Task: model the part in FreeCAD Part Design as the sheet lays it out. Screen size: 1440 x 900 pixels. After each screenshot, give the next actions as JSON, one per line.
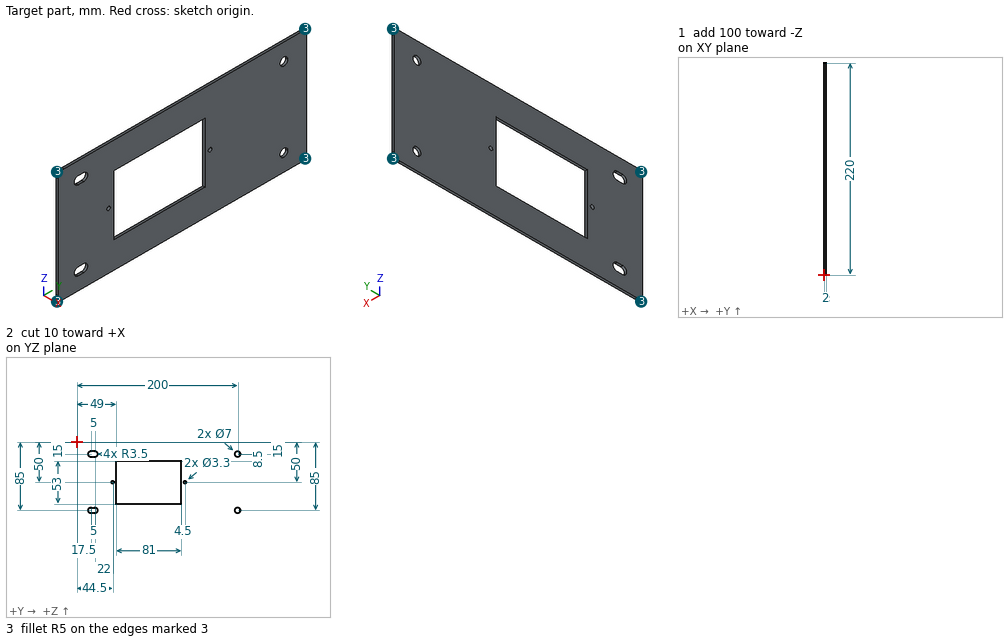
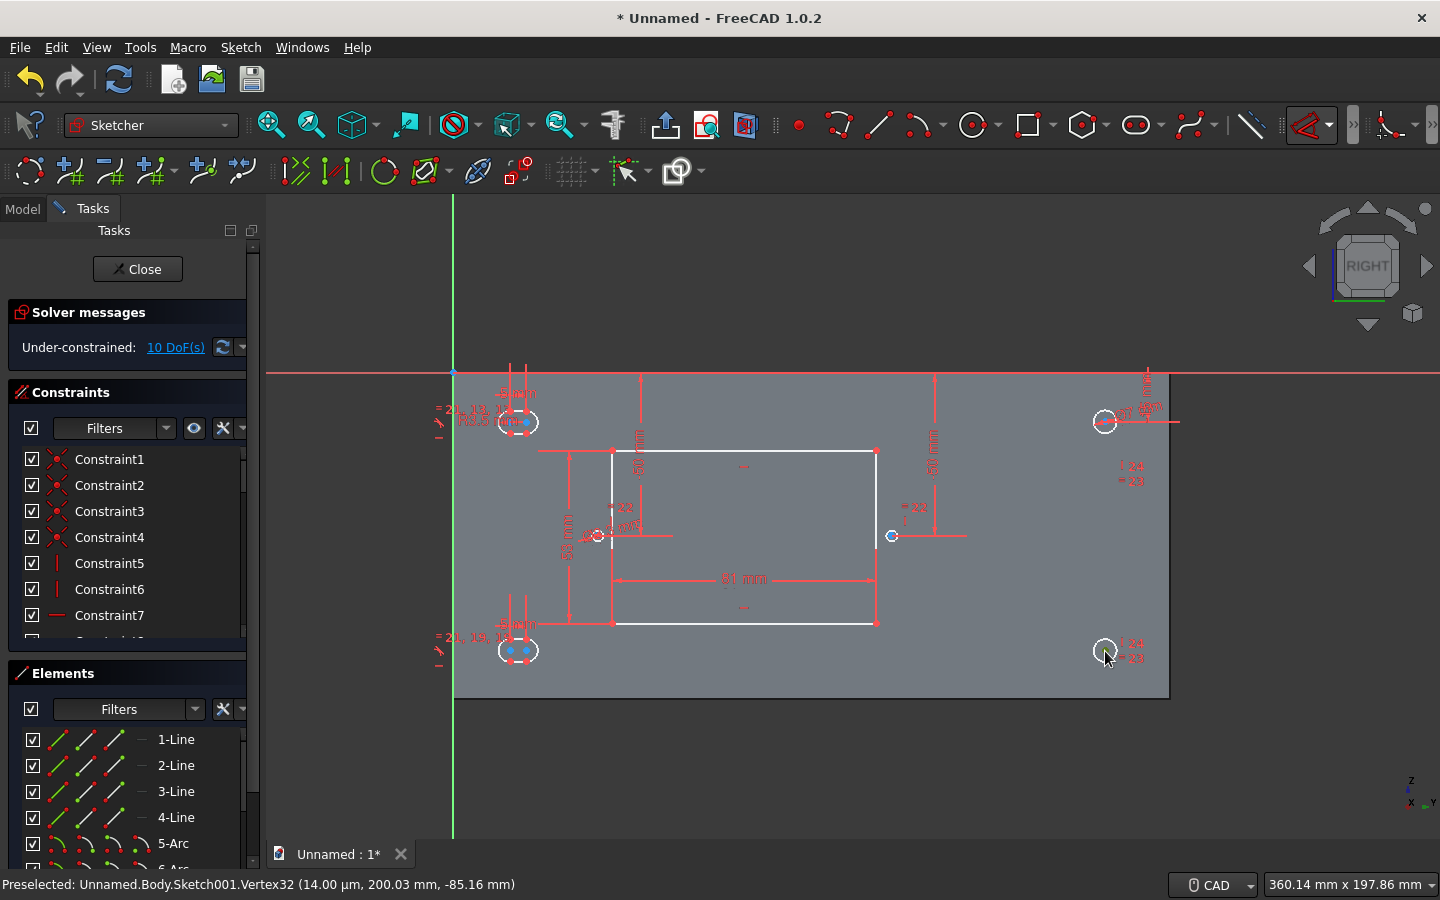
{"action": "key", "text": "i"}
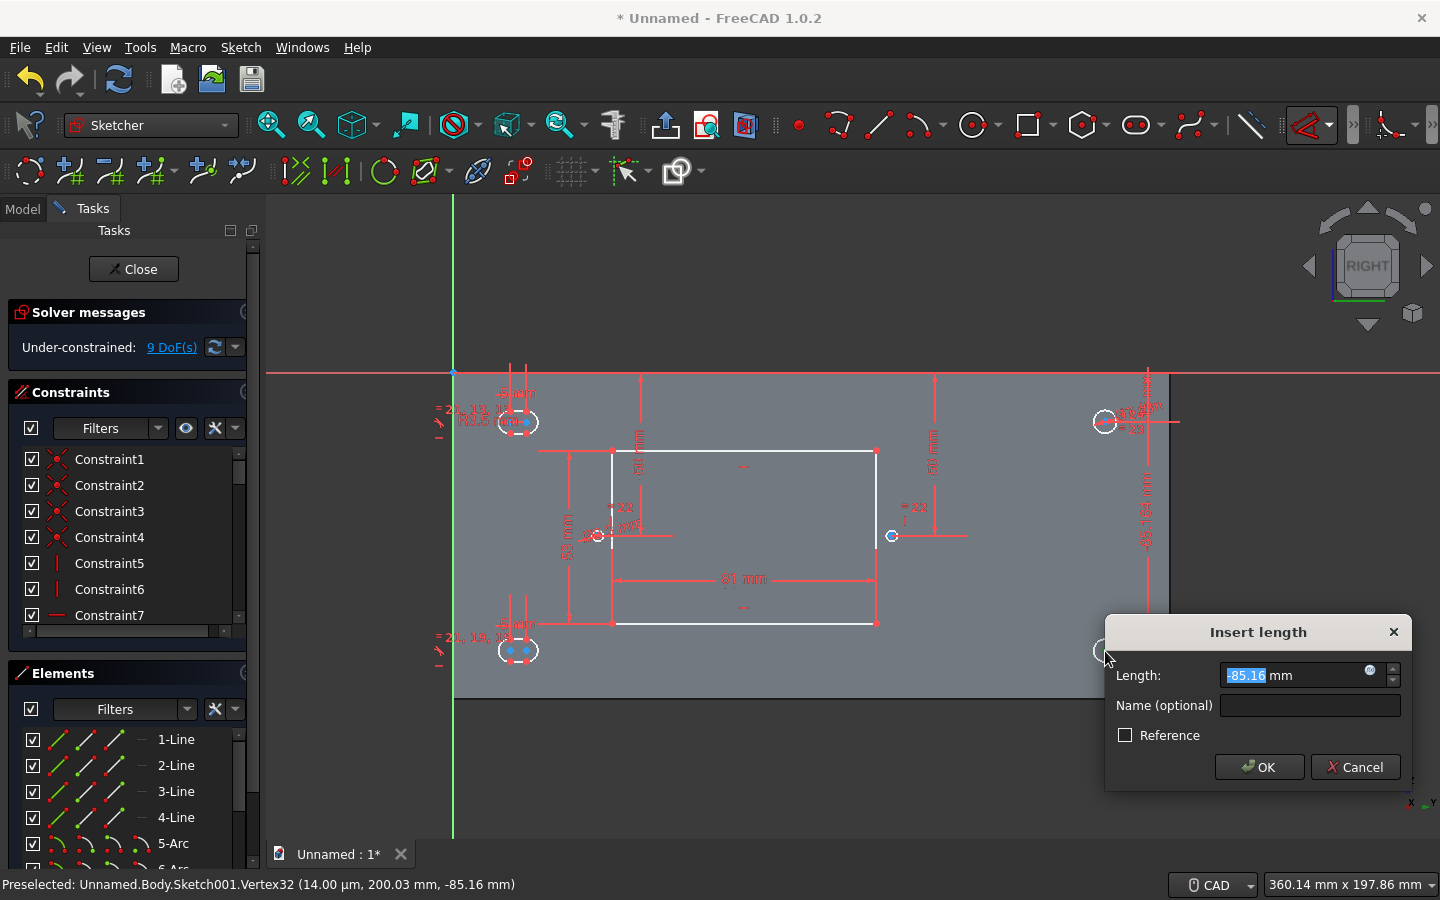
{"action": "type", "text": "-85"}
{"action": "key", "text": "Return"}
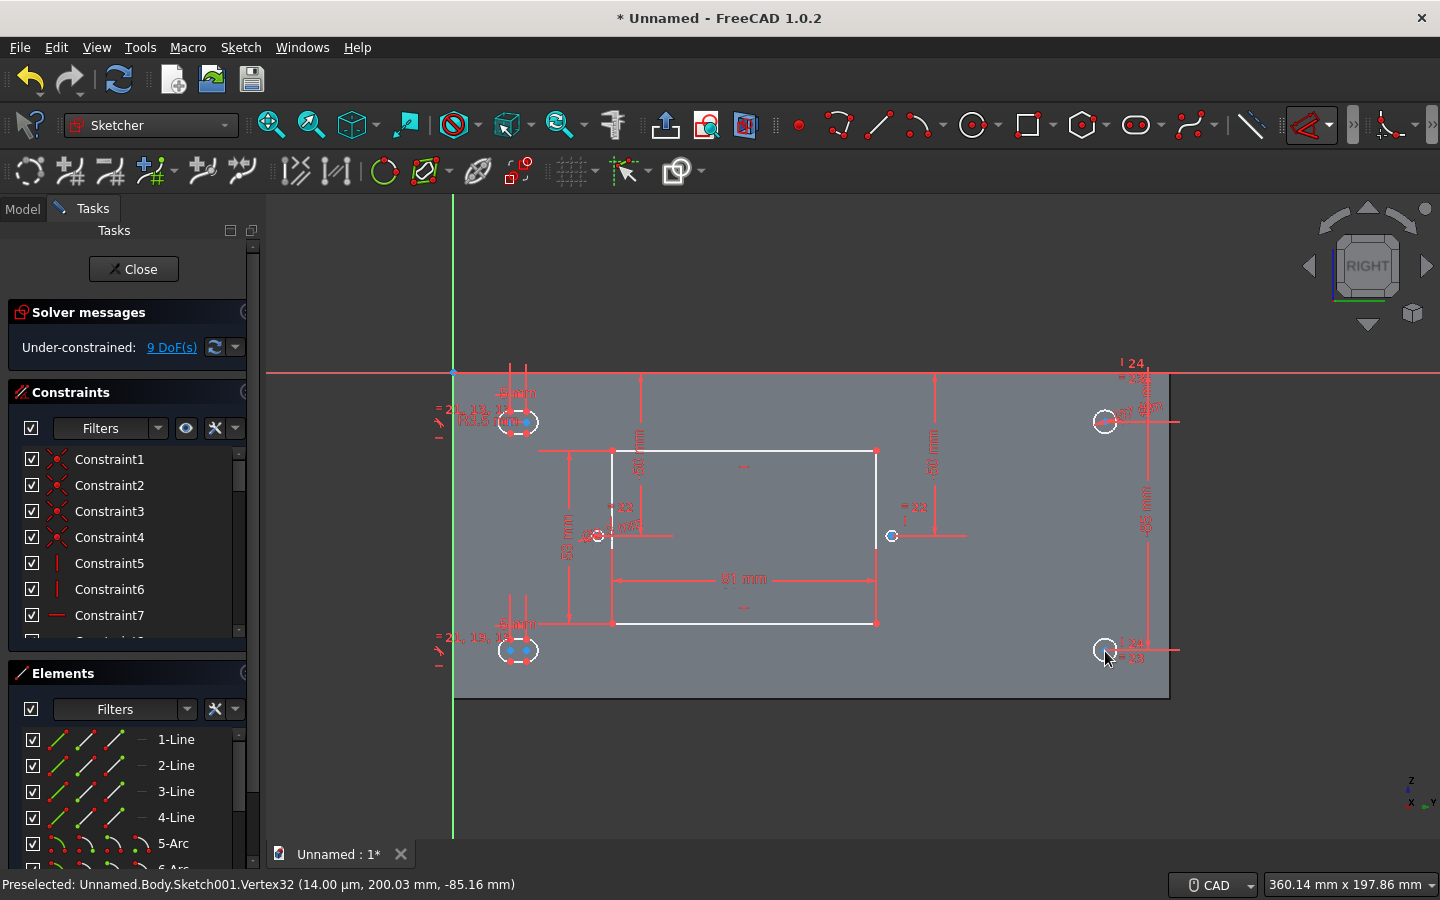
{"action": "left_click", "coordinate": [612, 451]}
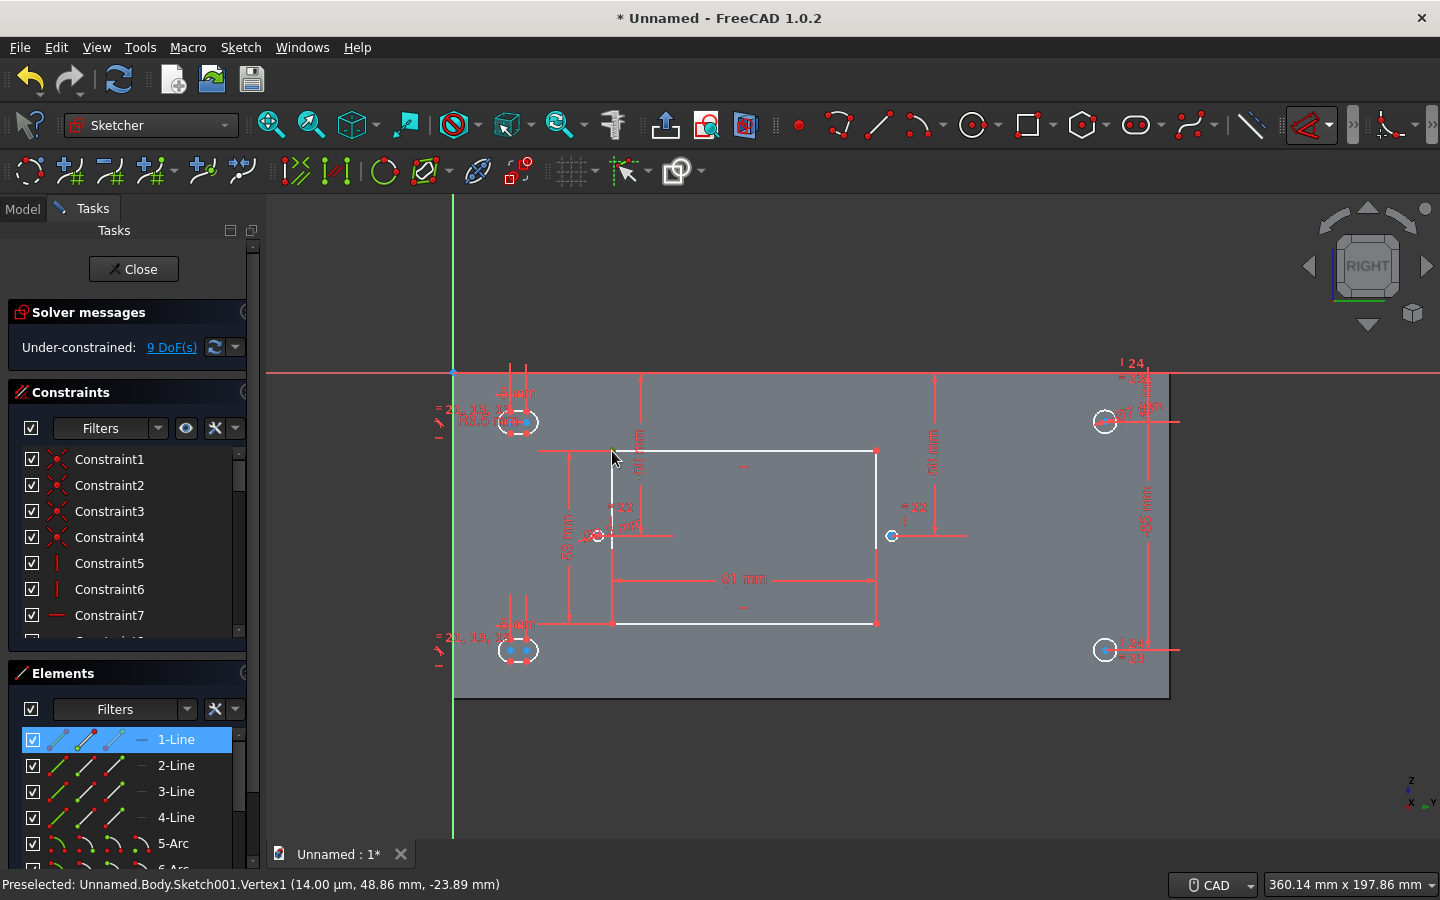
{"action": "left_click", "coordinate": [1332, 126]}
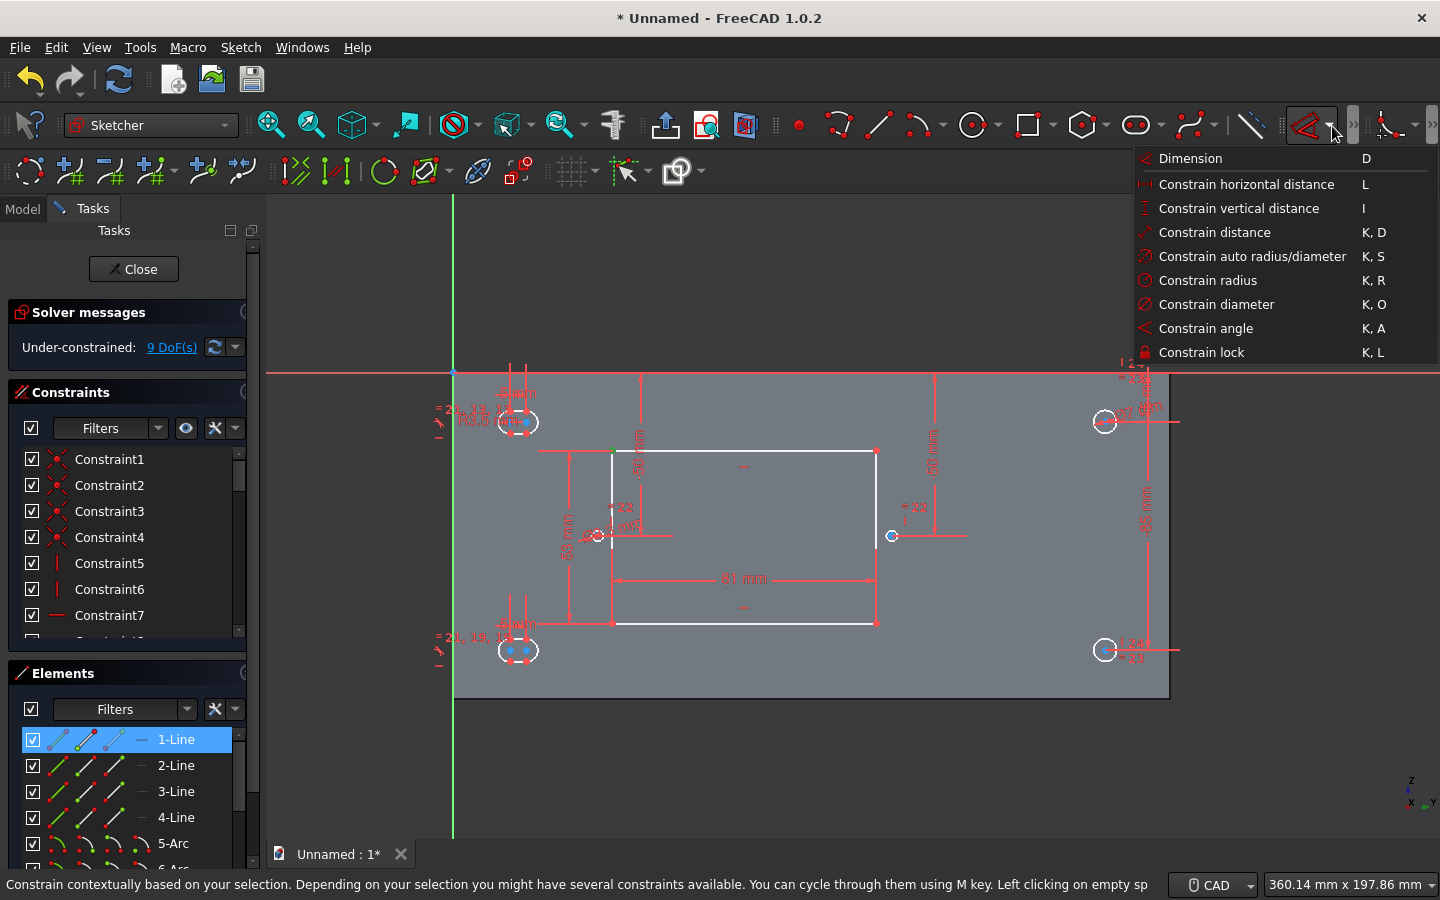
{"action": "left_click", "coordinate": [1286, 184]}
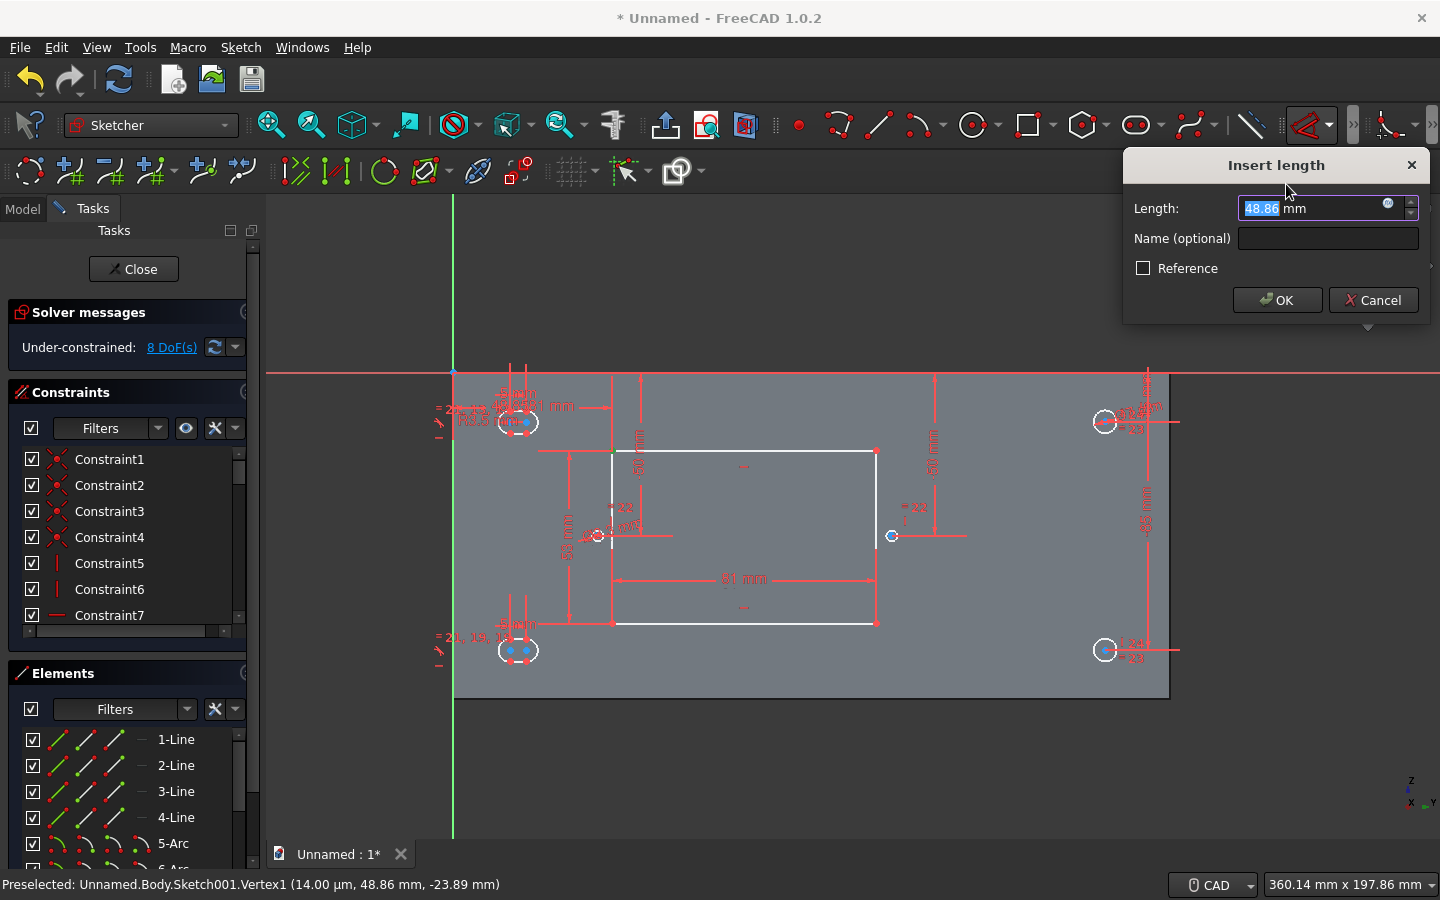
{"action": "type", "text": "49"}
{"action": "key", "text": "Return"}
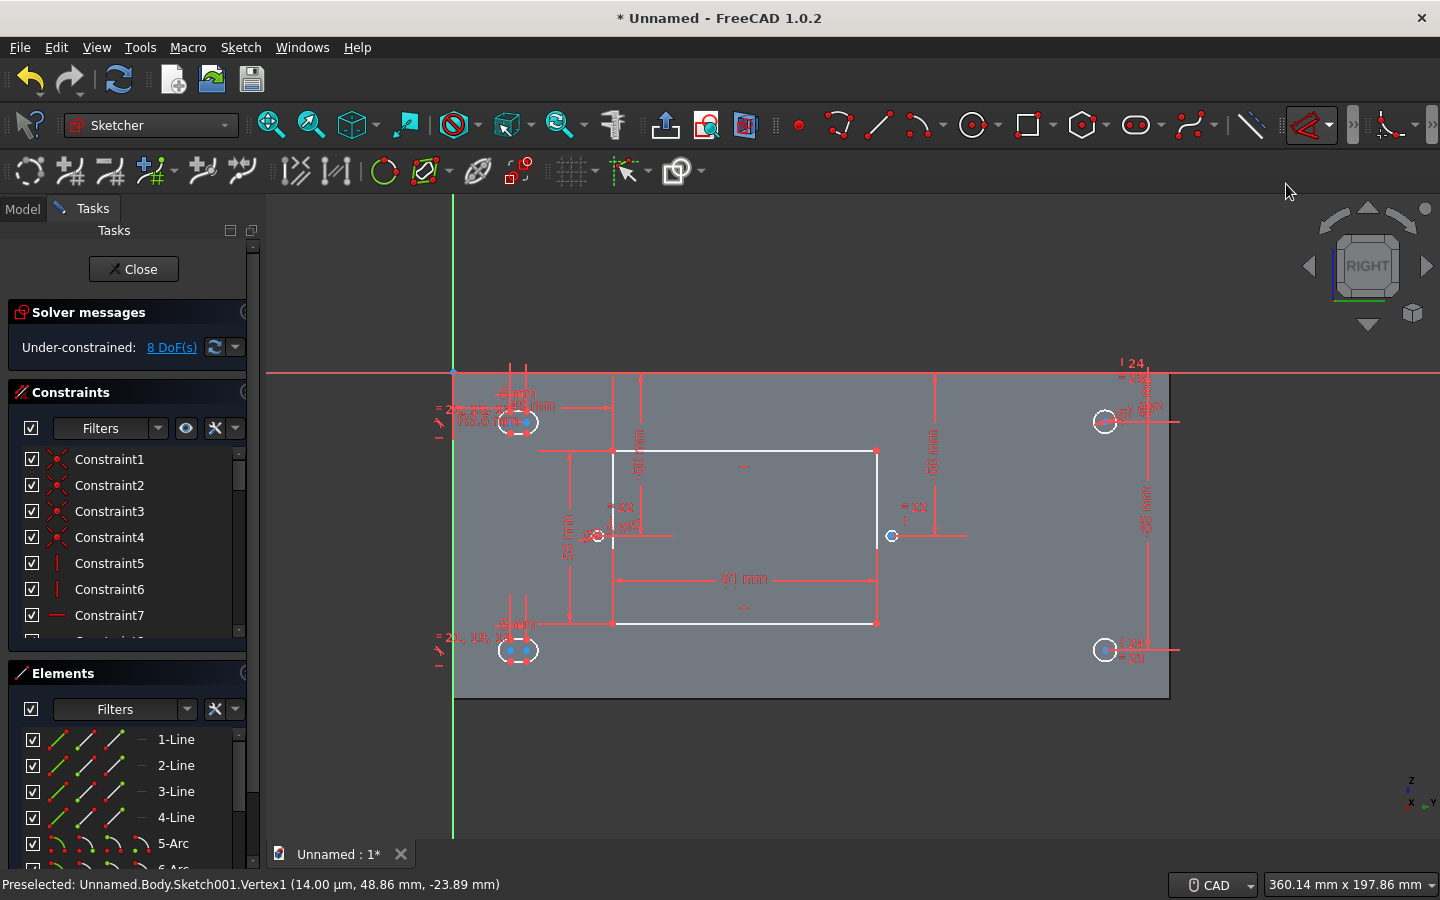
{"action": "left_click", "coordinate": [510, 422]}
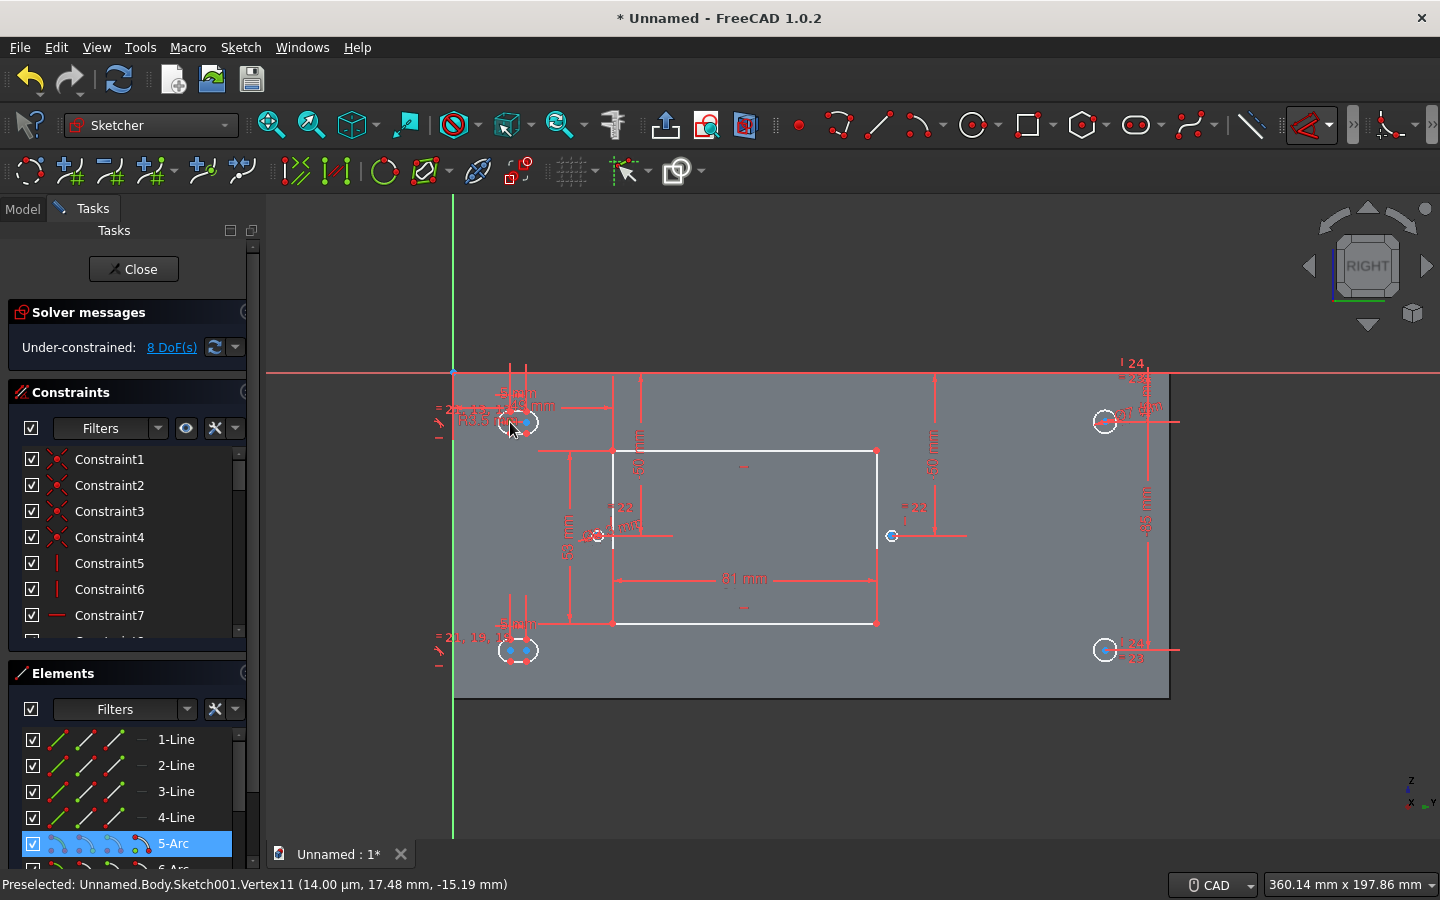
{"action": "key", "text": "i"}